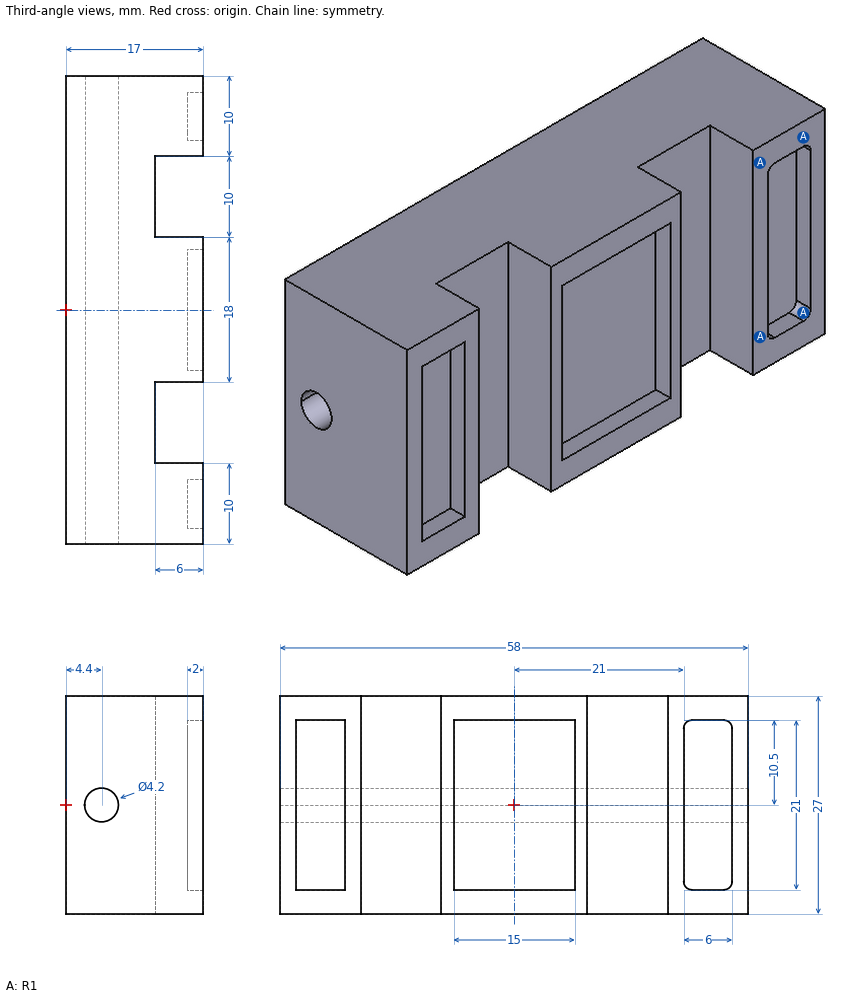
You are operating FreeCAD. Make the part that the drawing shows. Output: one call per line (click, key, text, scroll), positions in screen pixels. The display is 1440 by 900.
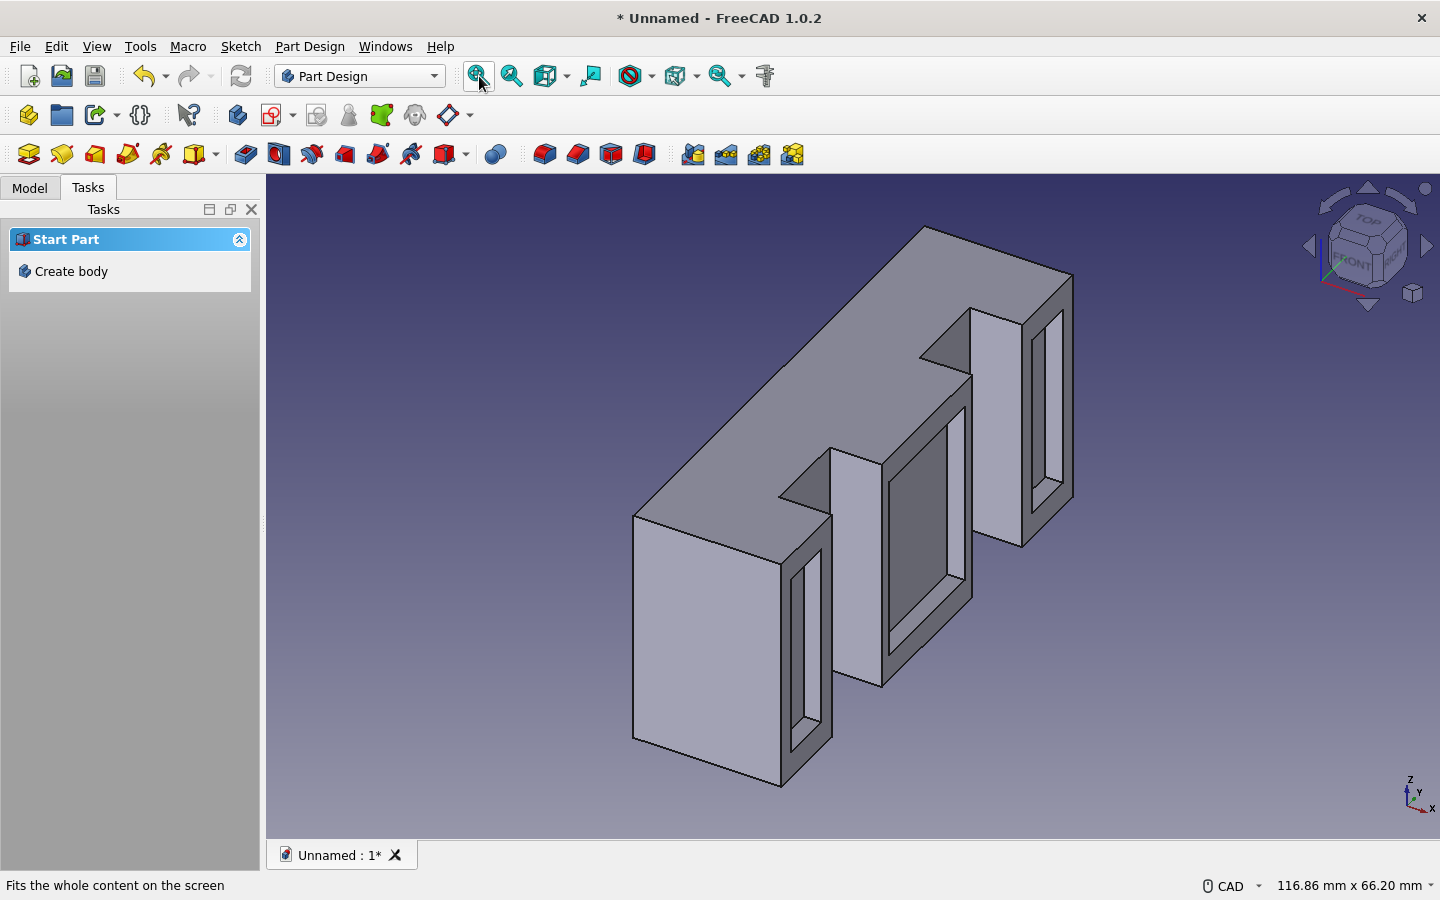
key(0)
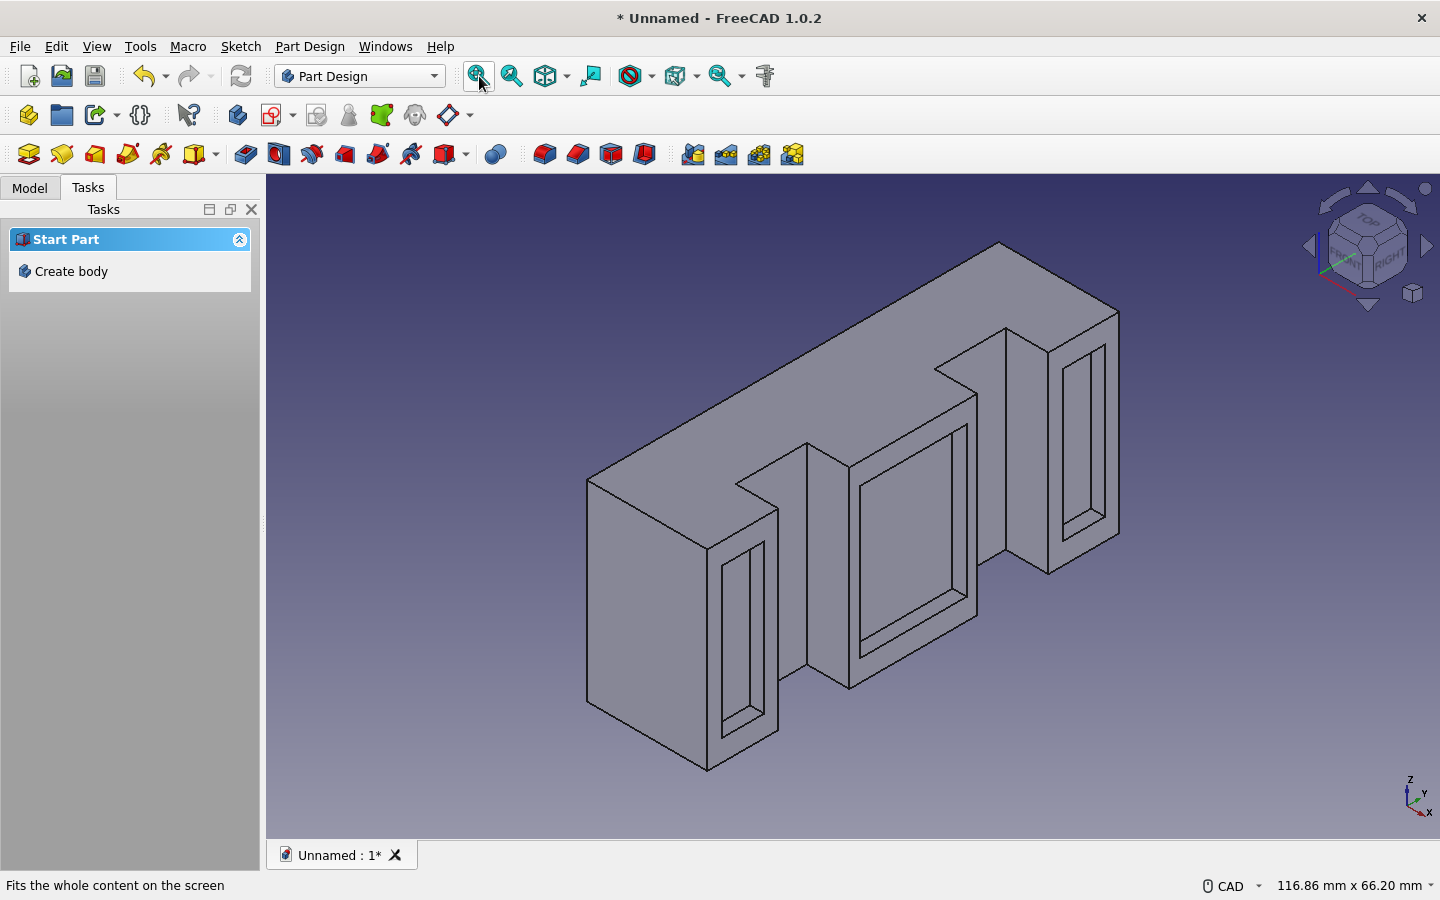
scroll(1098, 512, up, 4)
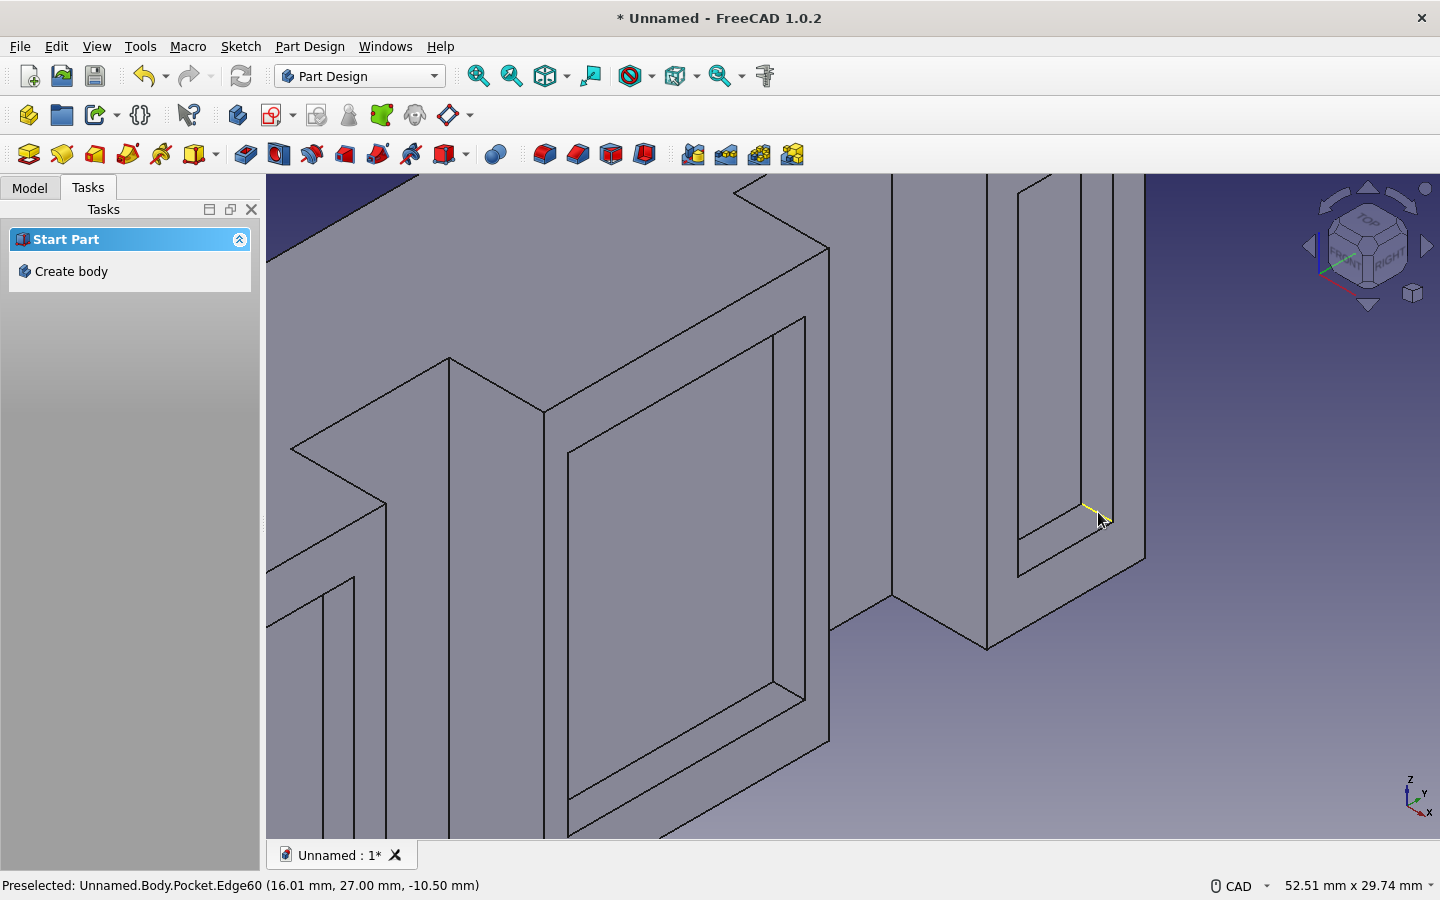
key(v)
key(f)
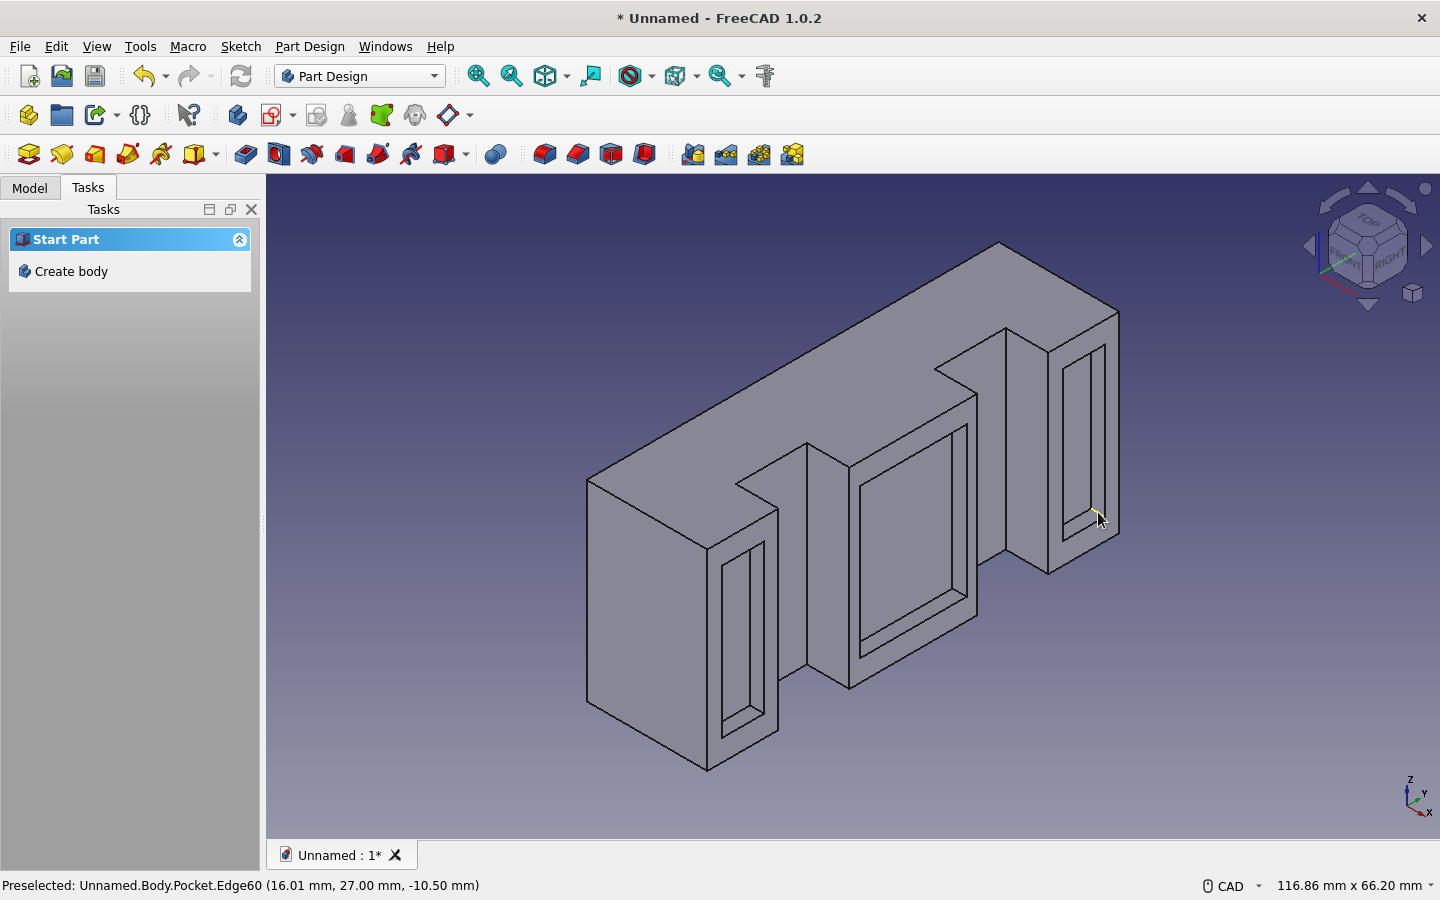
key(2)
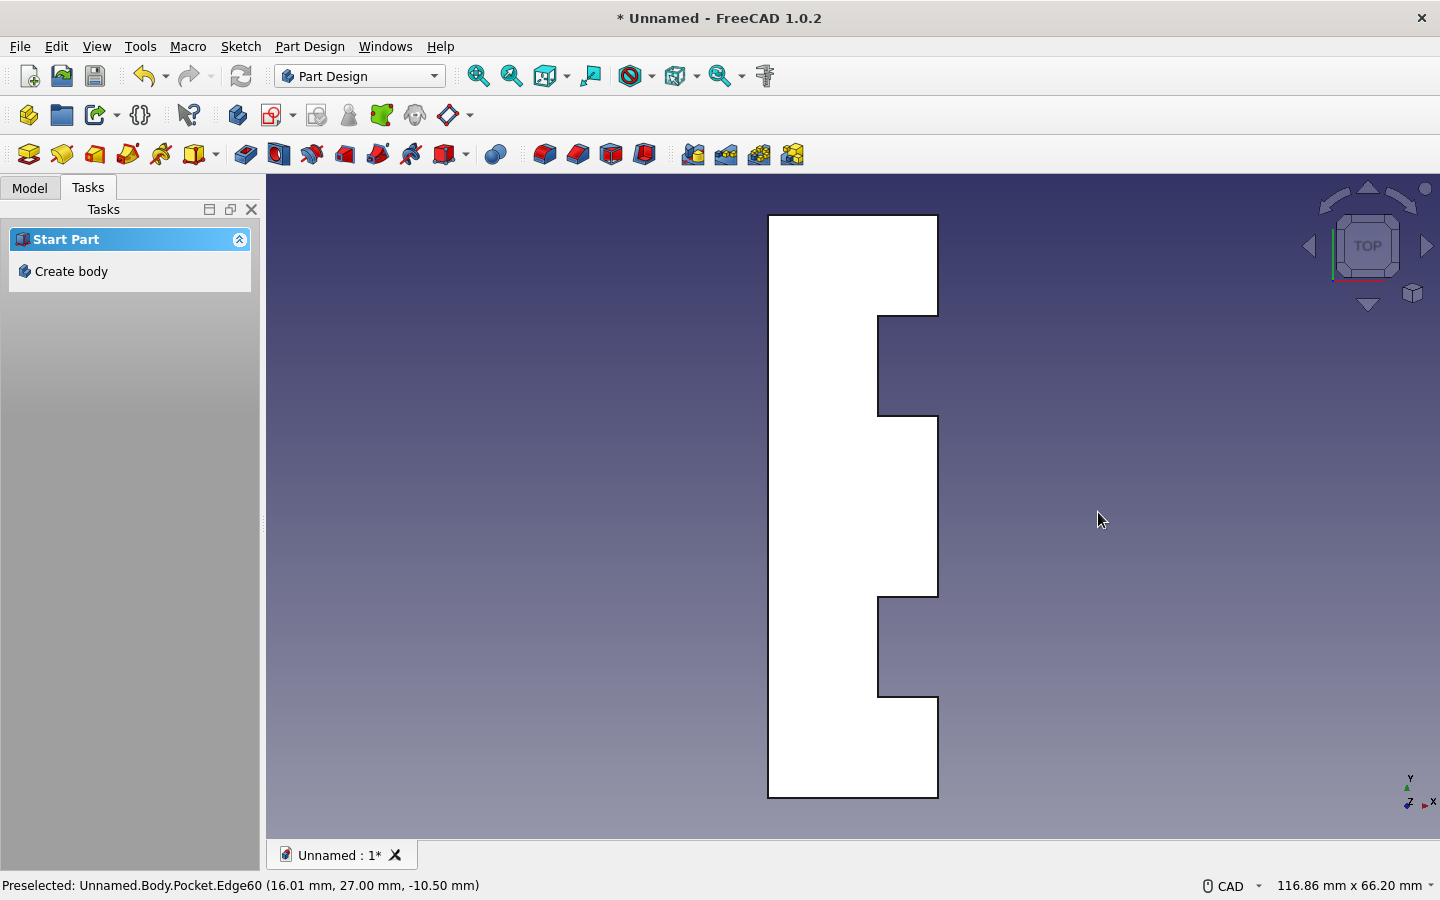
scroll(928, 234, up, 4)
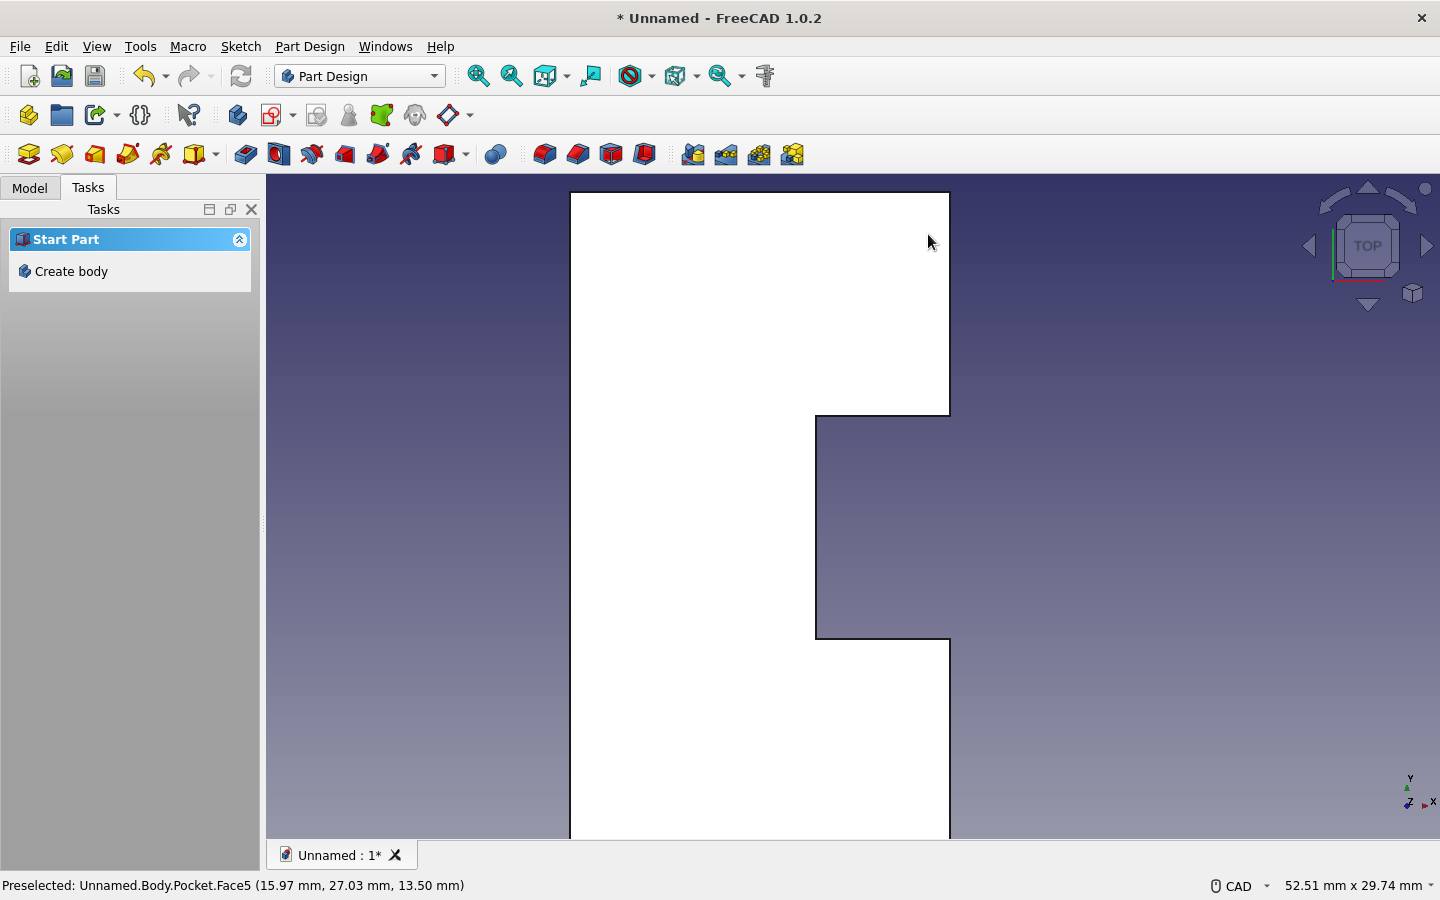
key(v)
key(f)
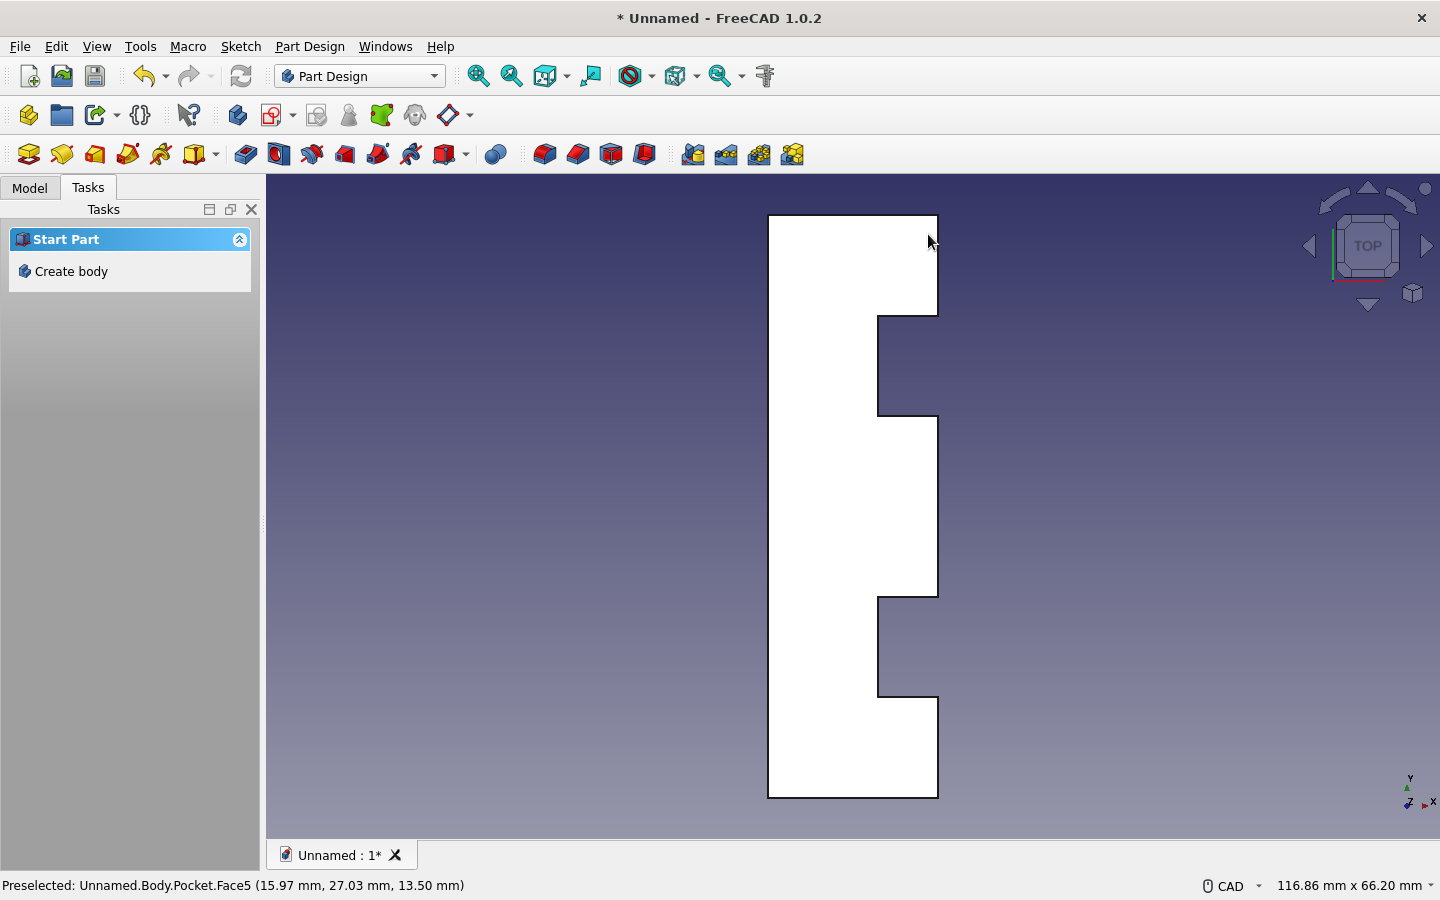
key(1)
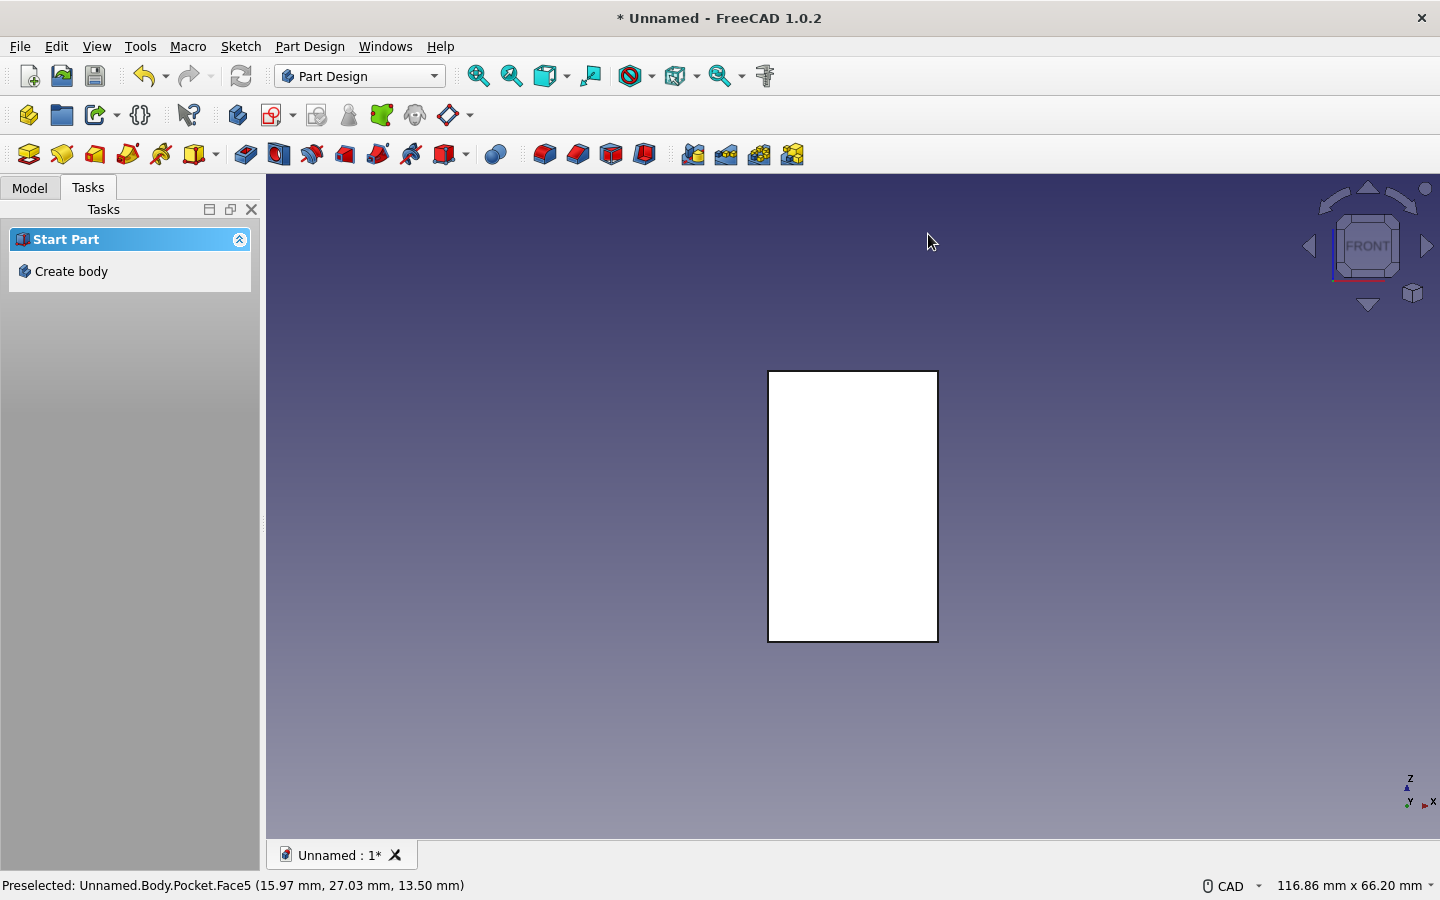
key(v)
key(f)